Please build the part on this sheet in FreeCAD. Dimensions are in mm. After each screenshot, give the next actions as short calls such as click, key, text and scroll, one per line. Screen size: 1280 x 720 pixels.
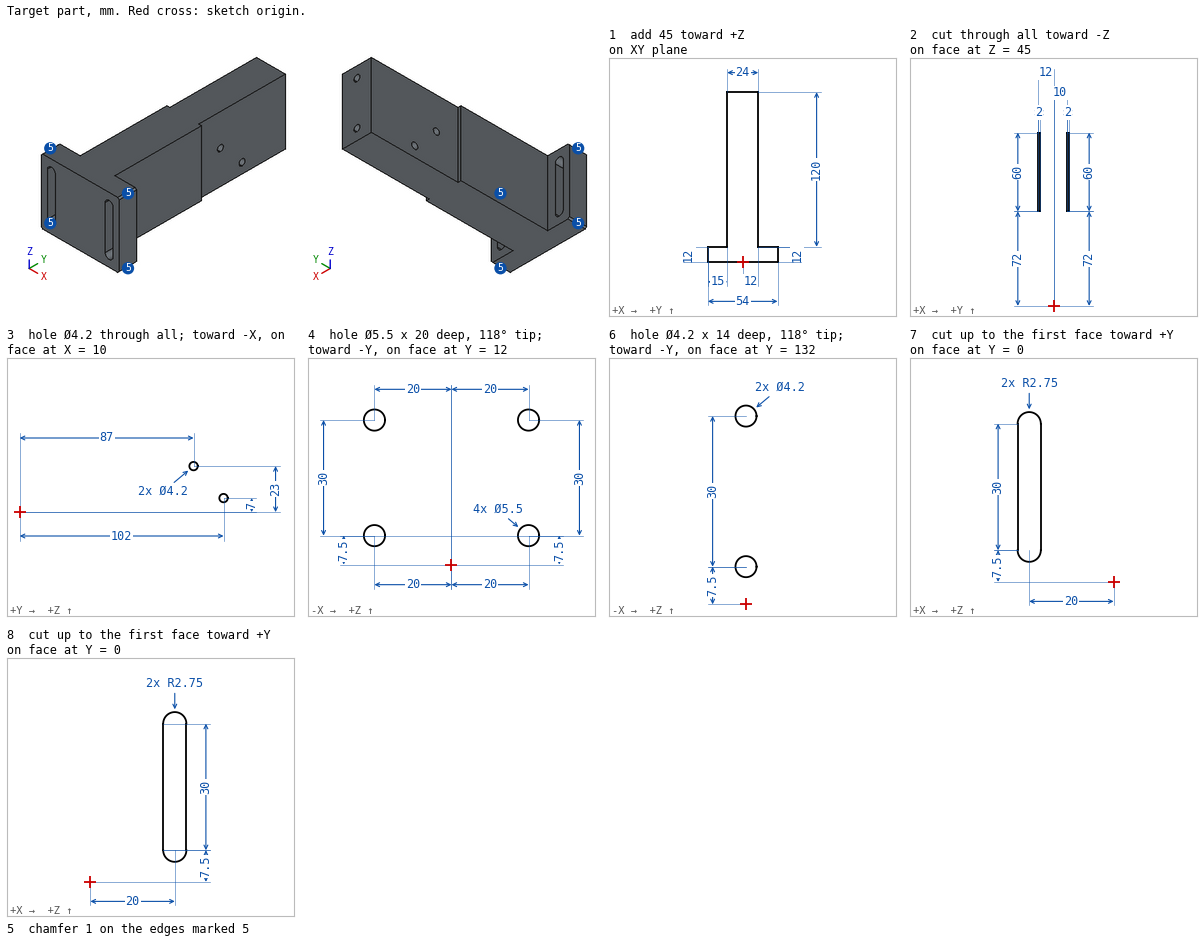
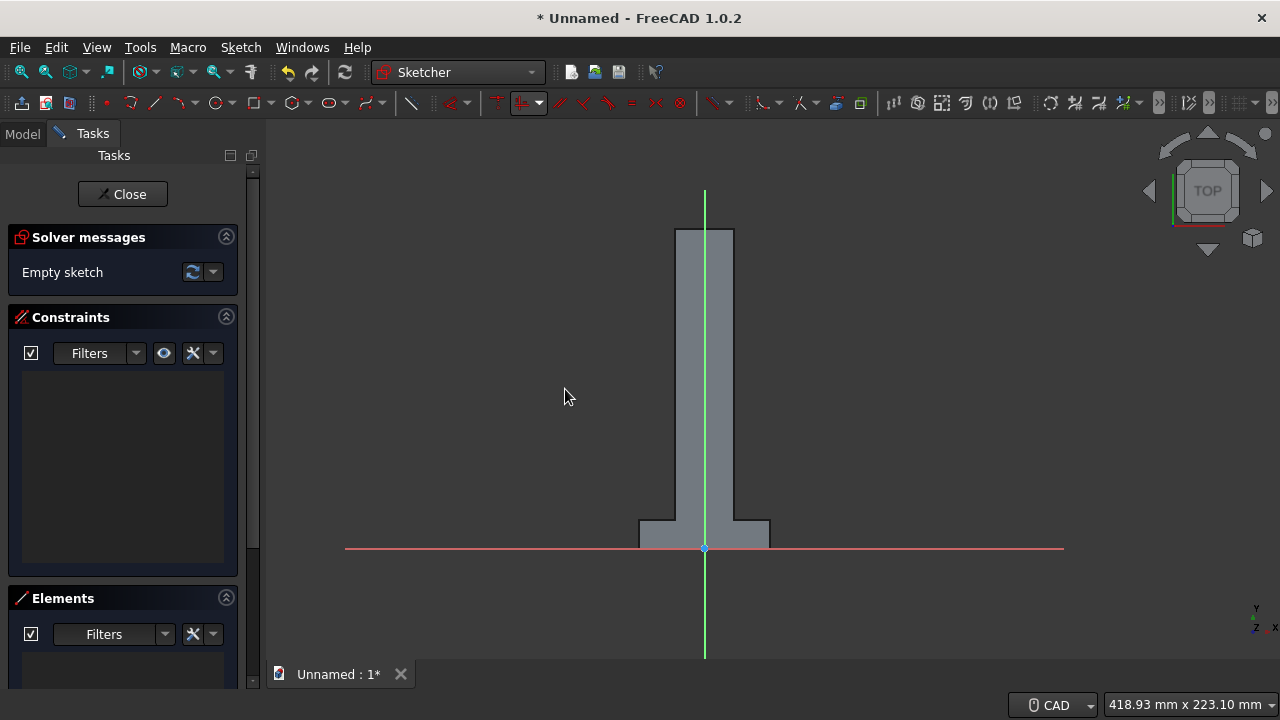
click(254, 104)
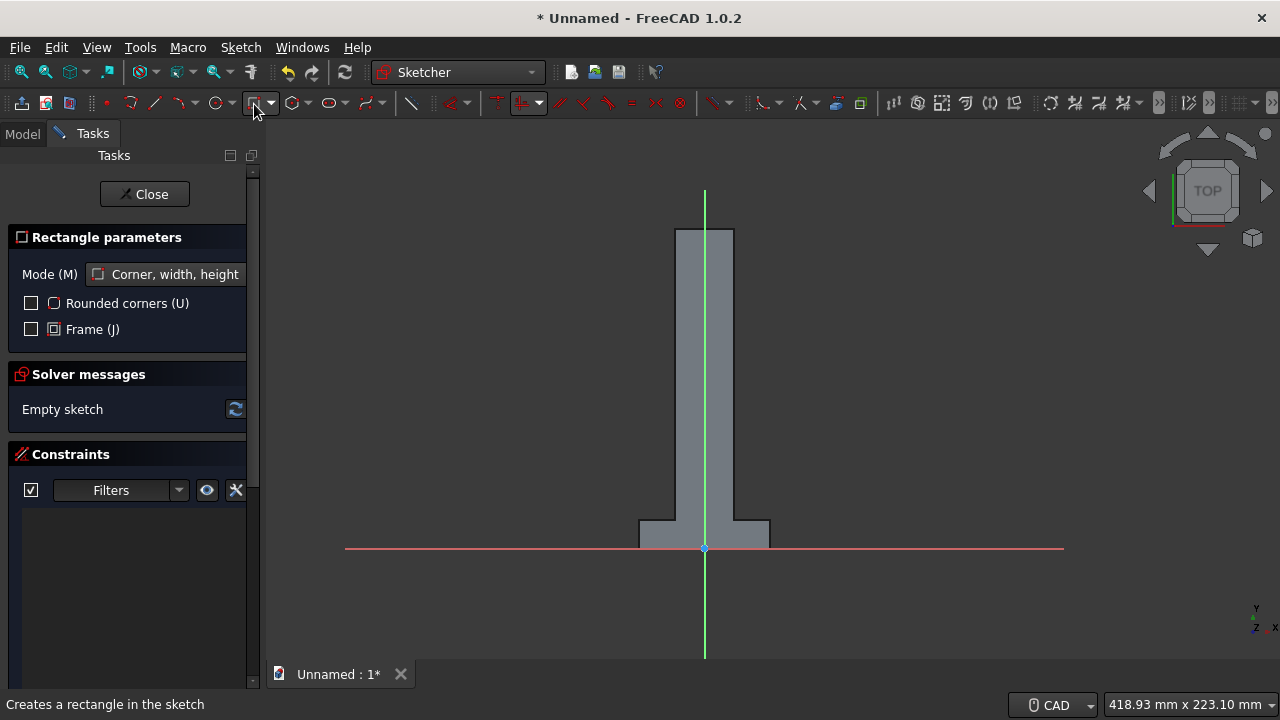
scroll(675, 229, up, 6)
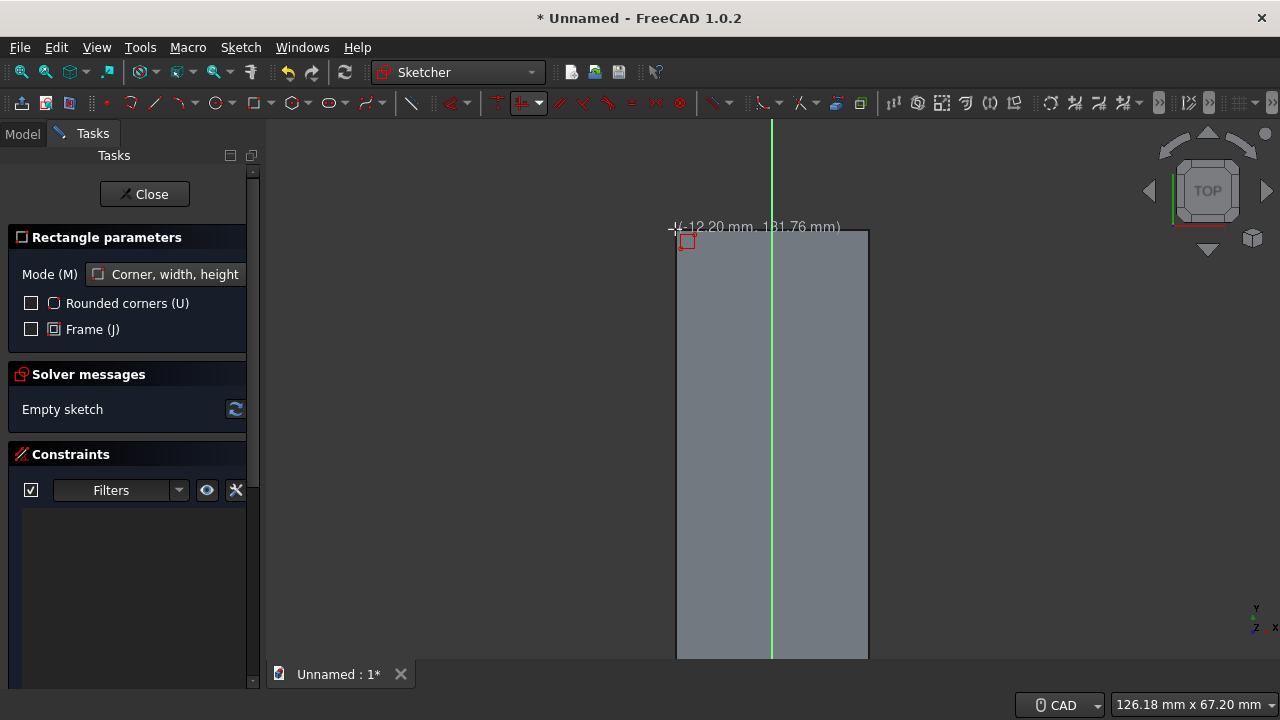
click(676, 230)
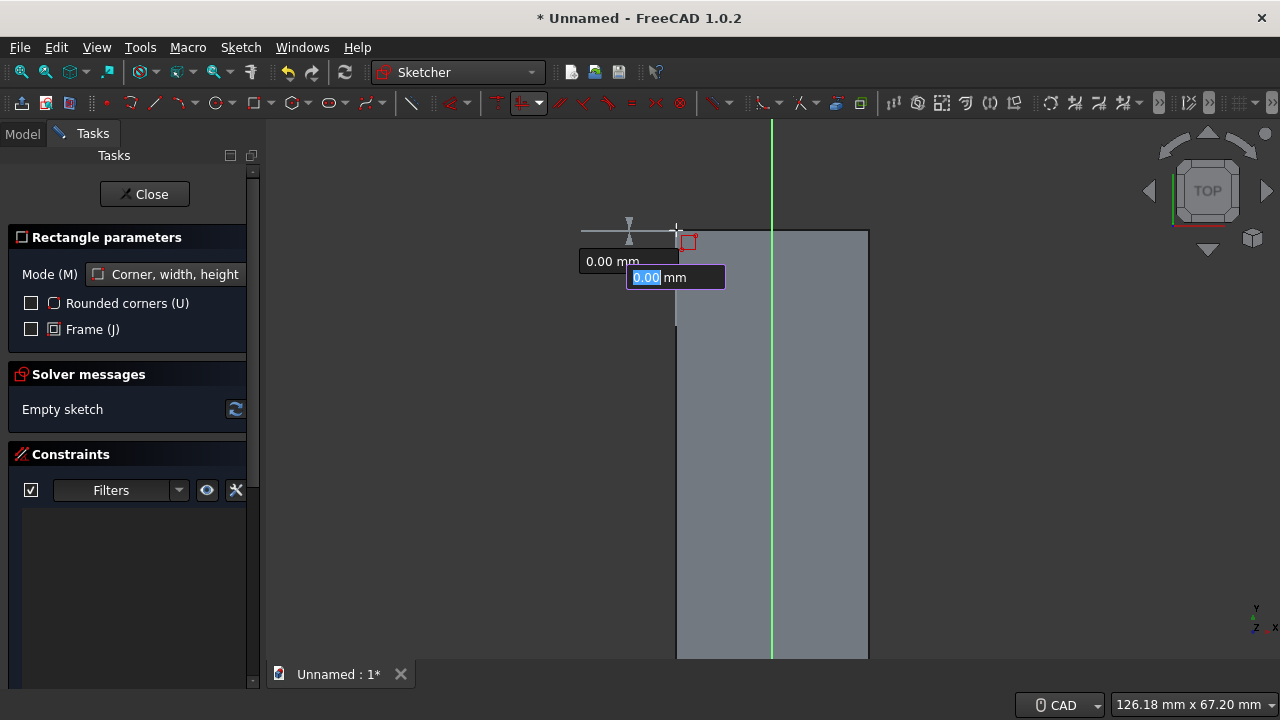
scroll(675, 229, down, 6)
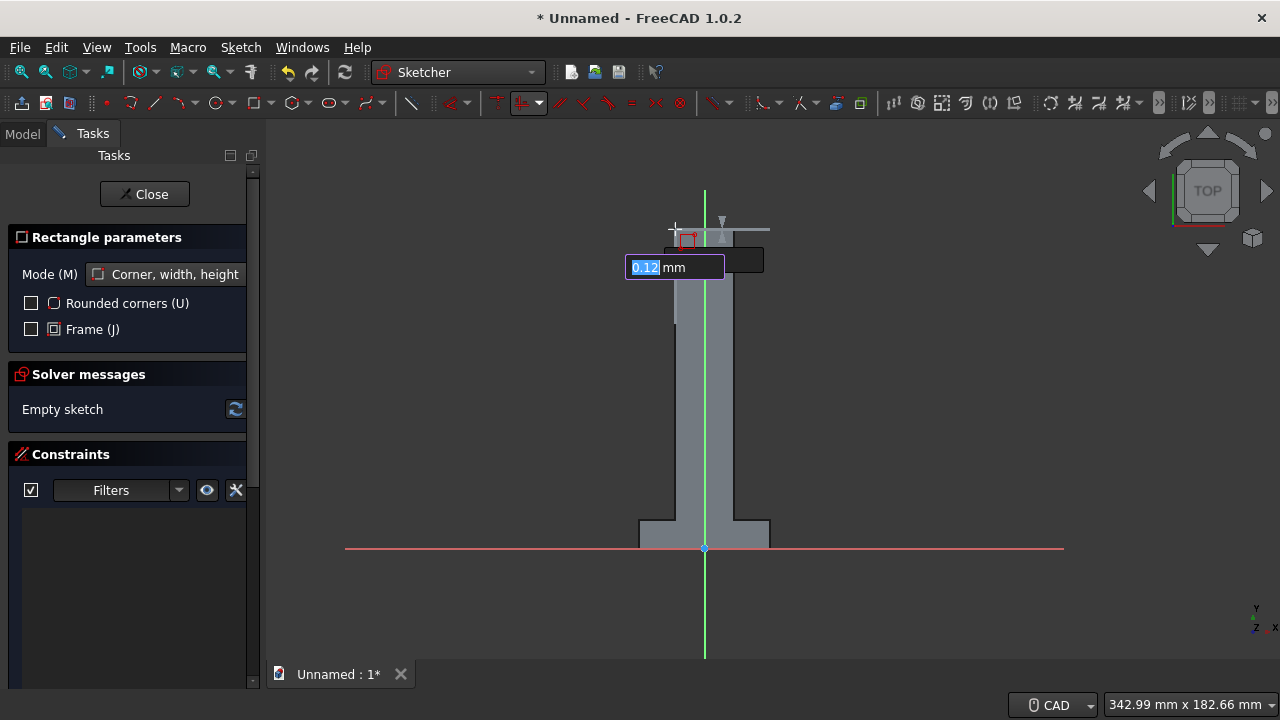
click(680, 375)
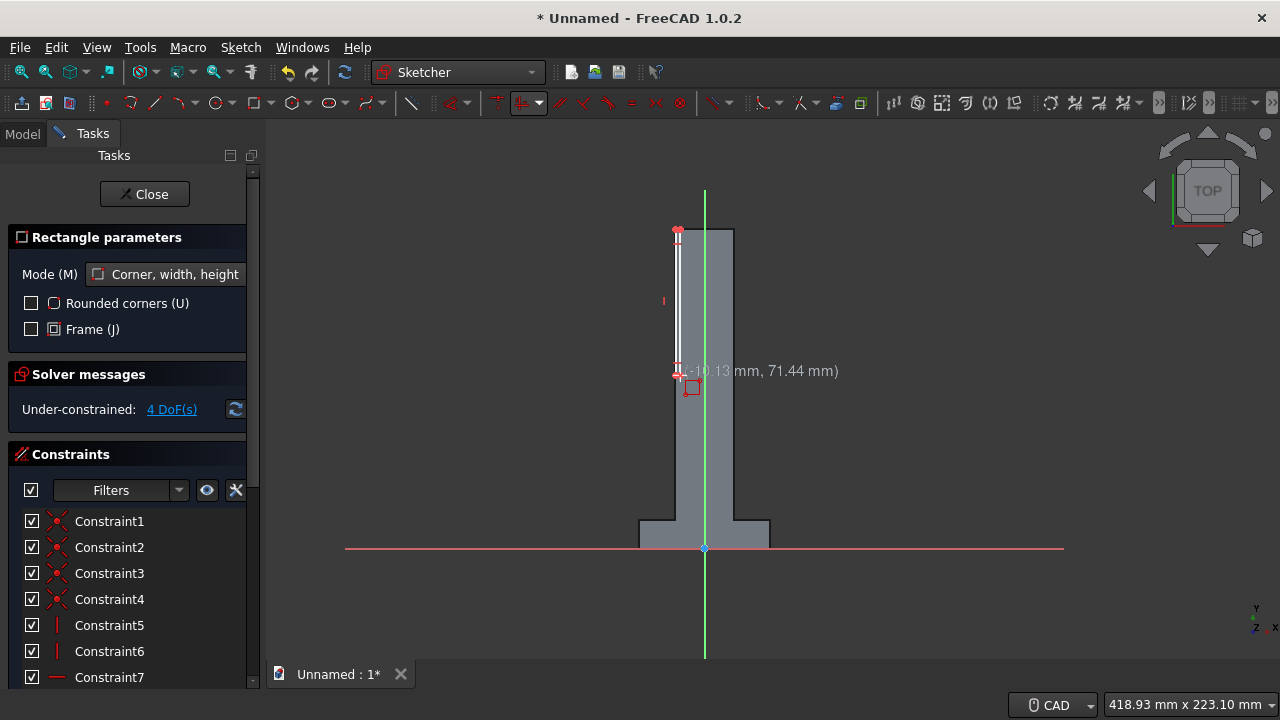
scroll(729, 229, up, 6)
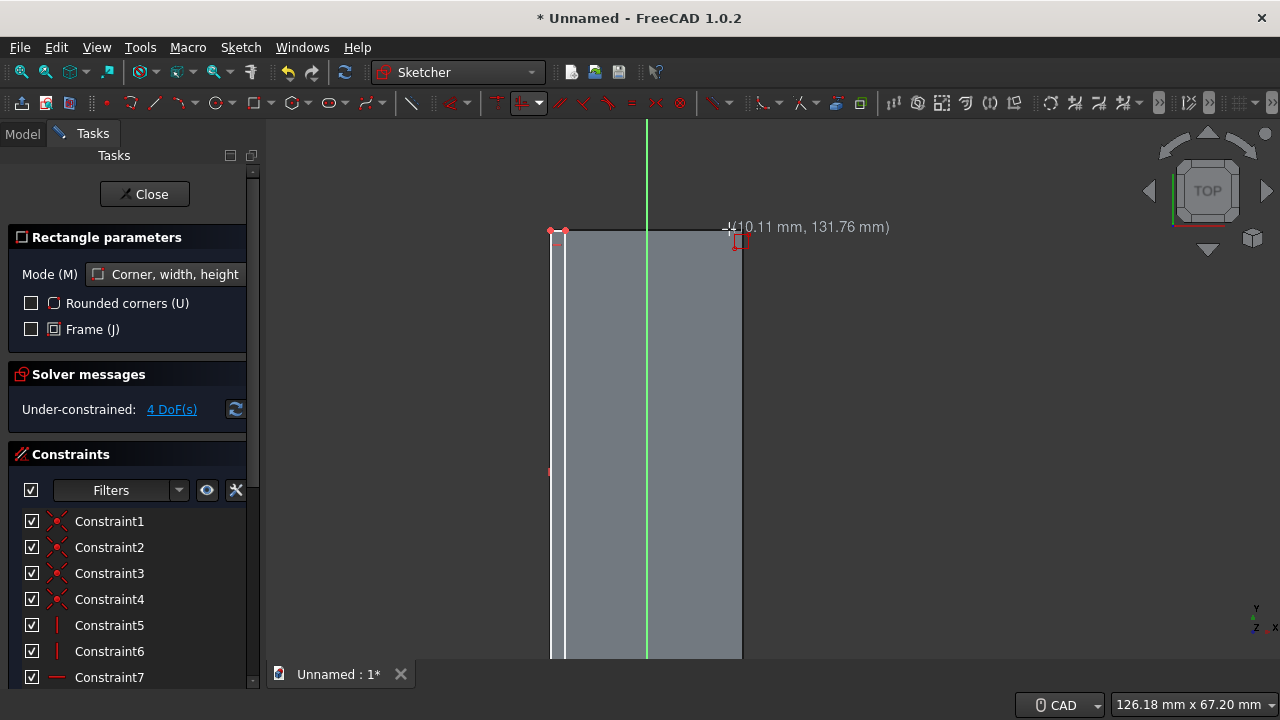
click(727, 230)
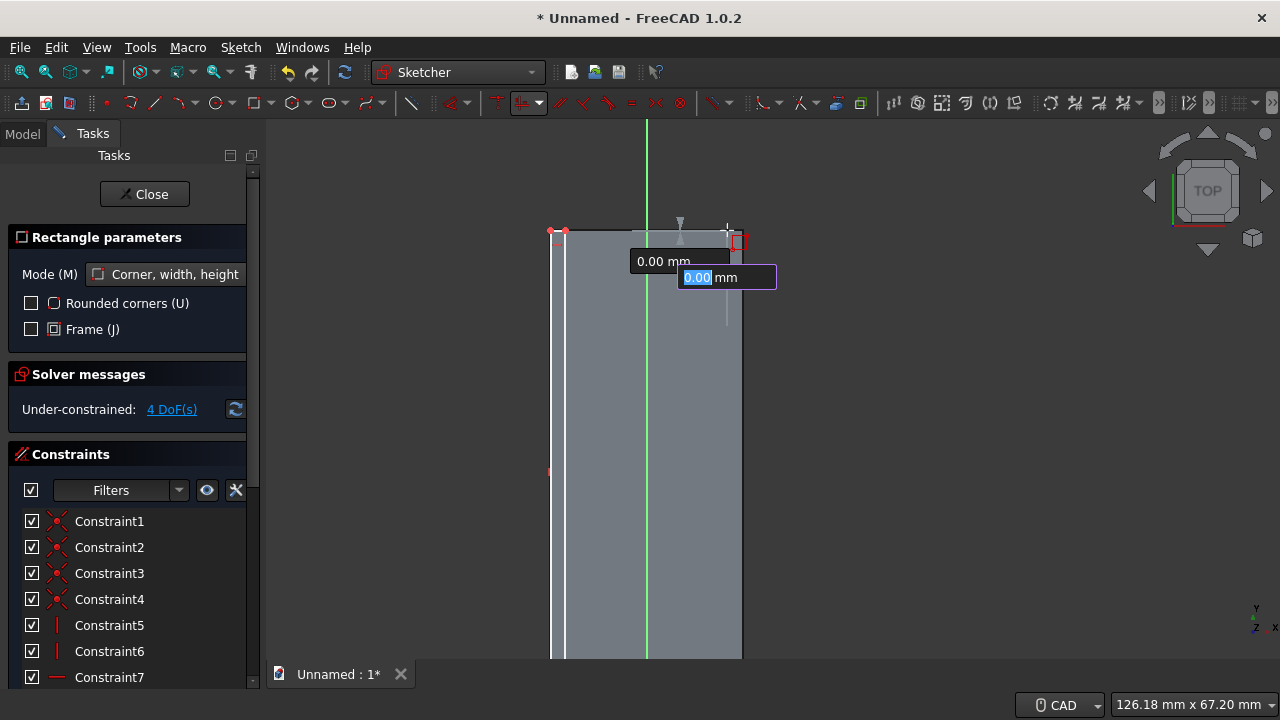
scroll(729, 229, down, 6)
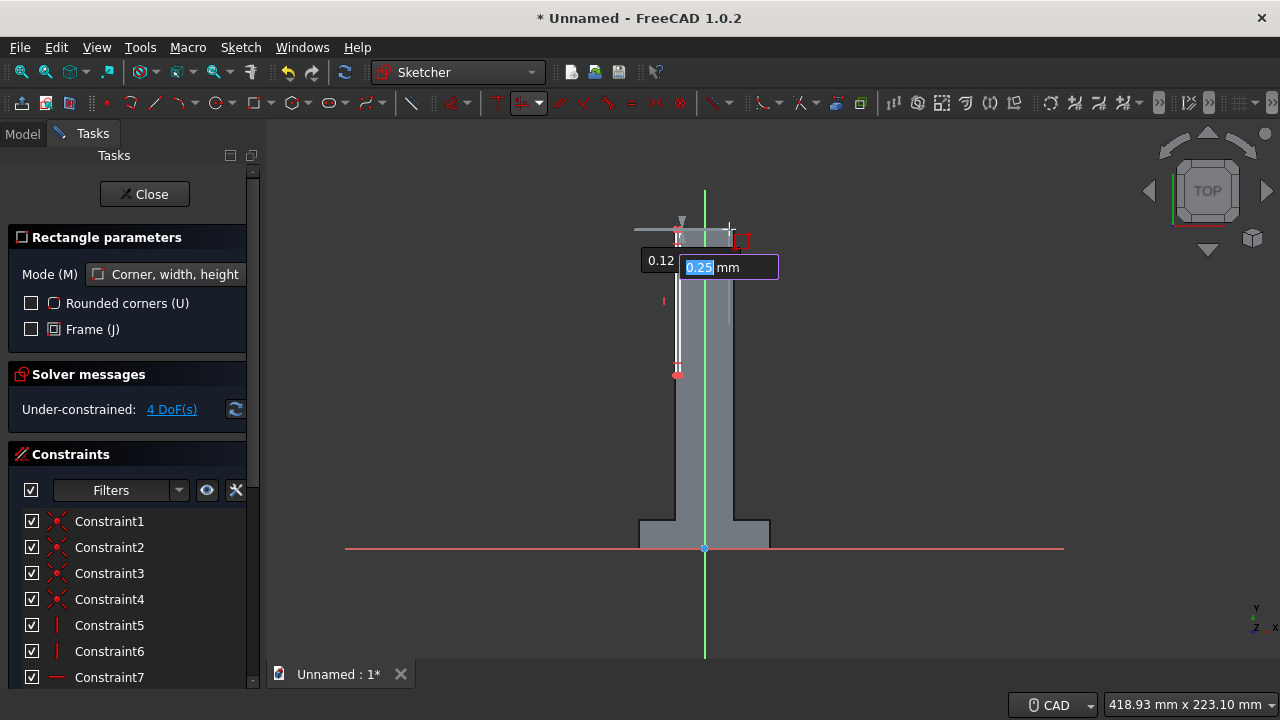
click(734, 375)
key(Escape)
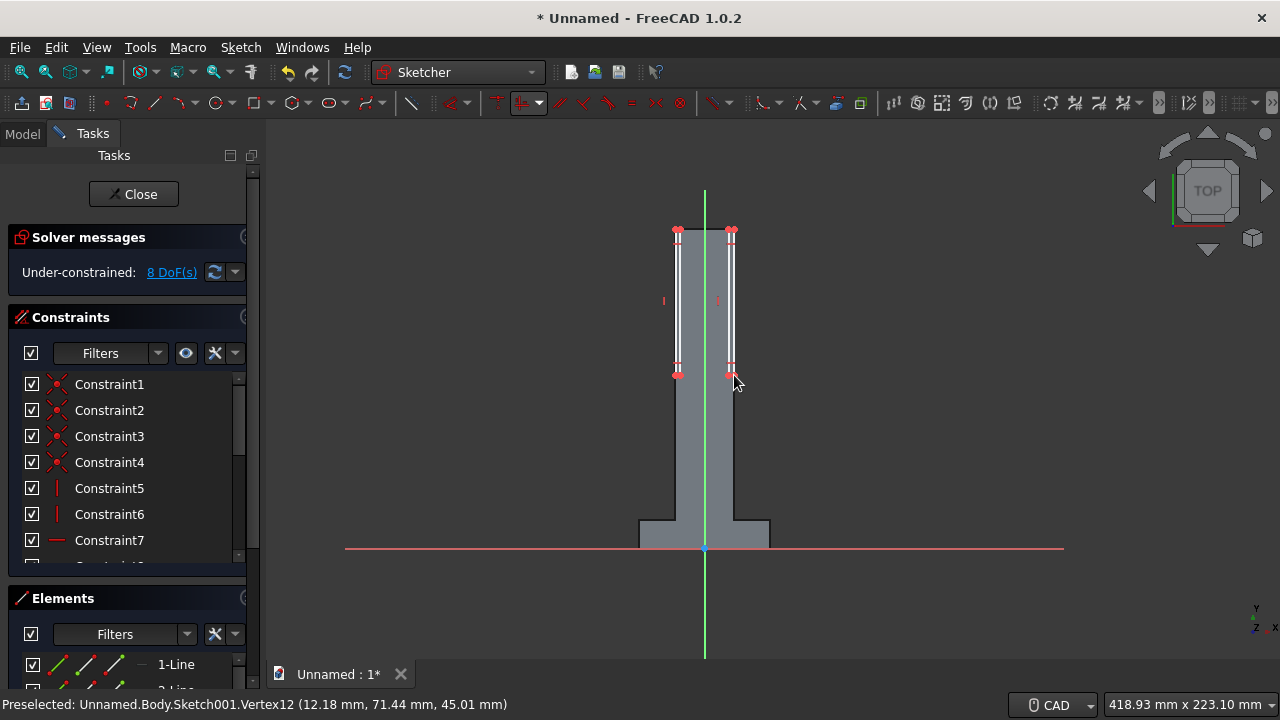
click(450, 104)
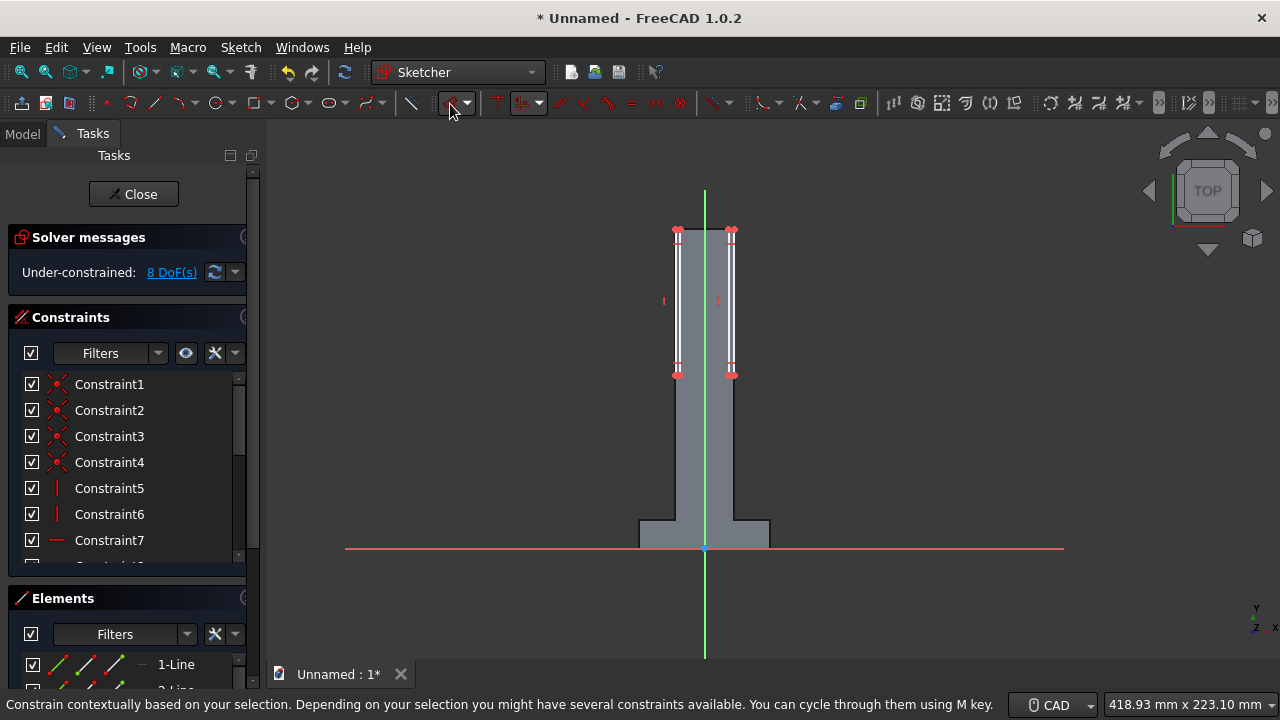
scroll(678, 376, up, 11)